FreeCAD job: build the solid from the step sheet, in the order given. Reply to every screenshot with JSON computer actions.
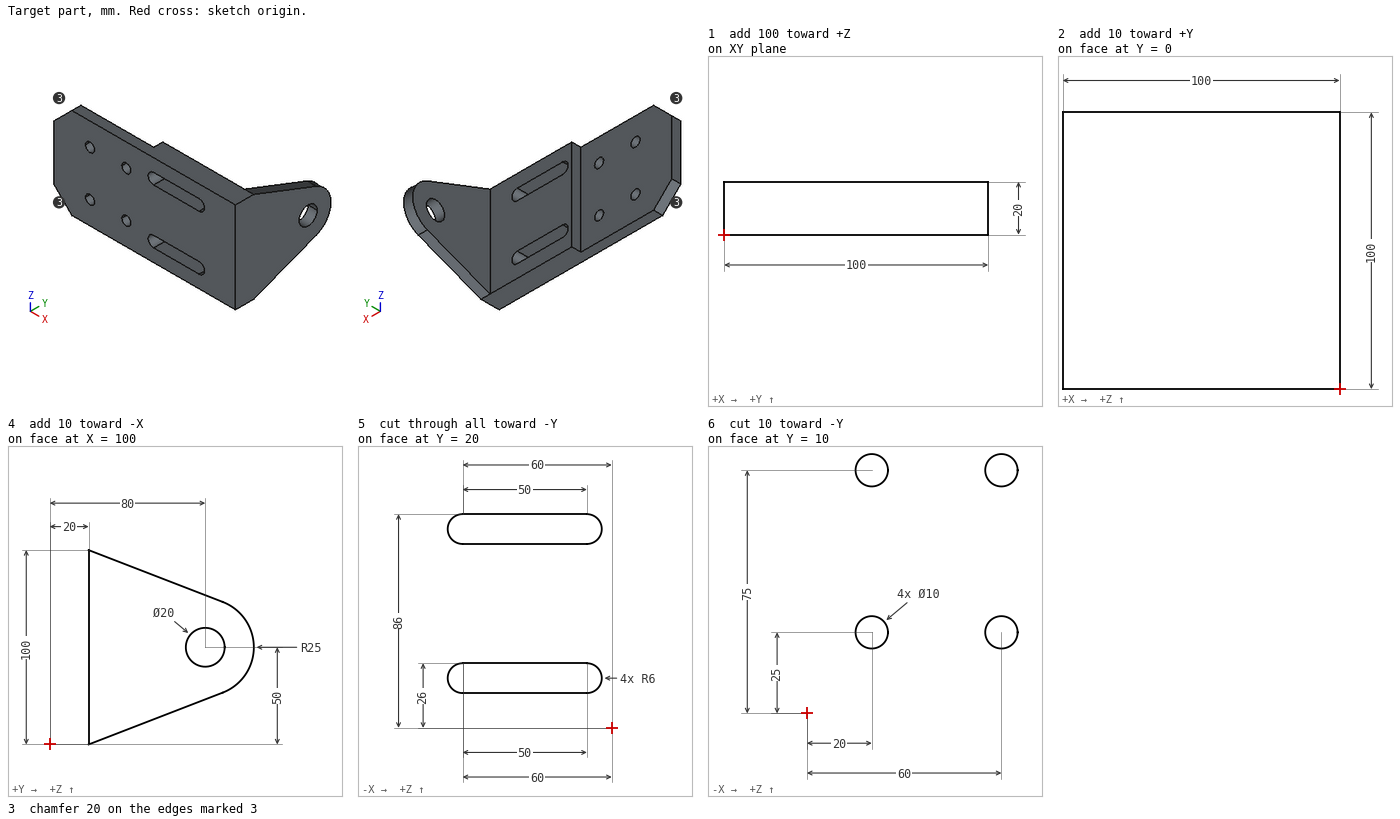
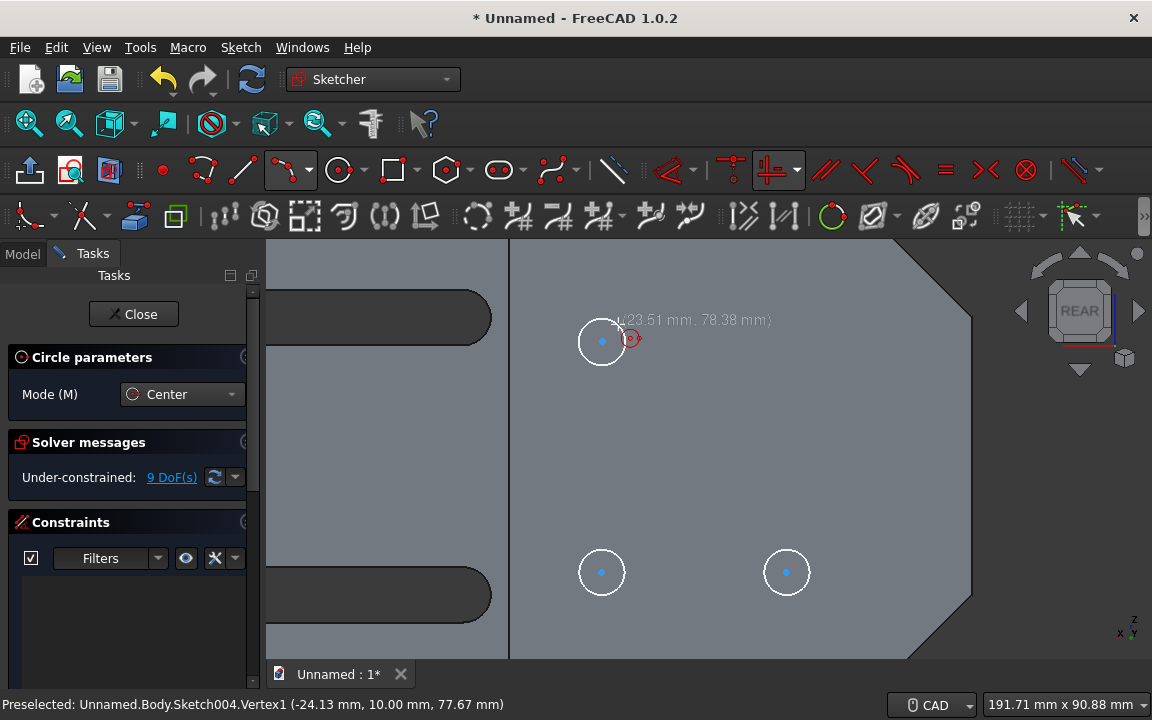
{"action": "left_click", "coordinate": [787, 341]}
{"action": "left_click", "coordinate": [803, 324]}
{"action": "key", "text": "Escape"}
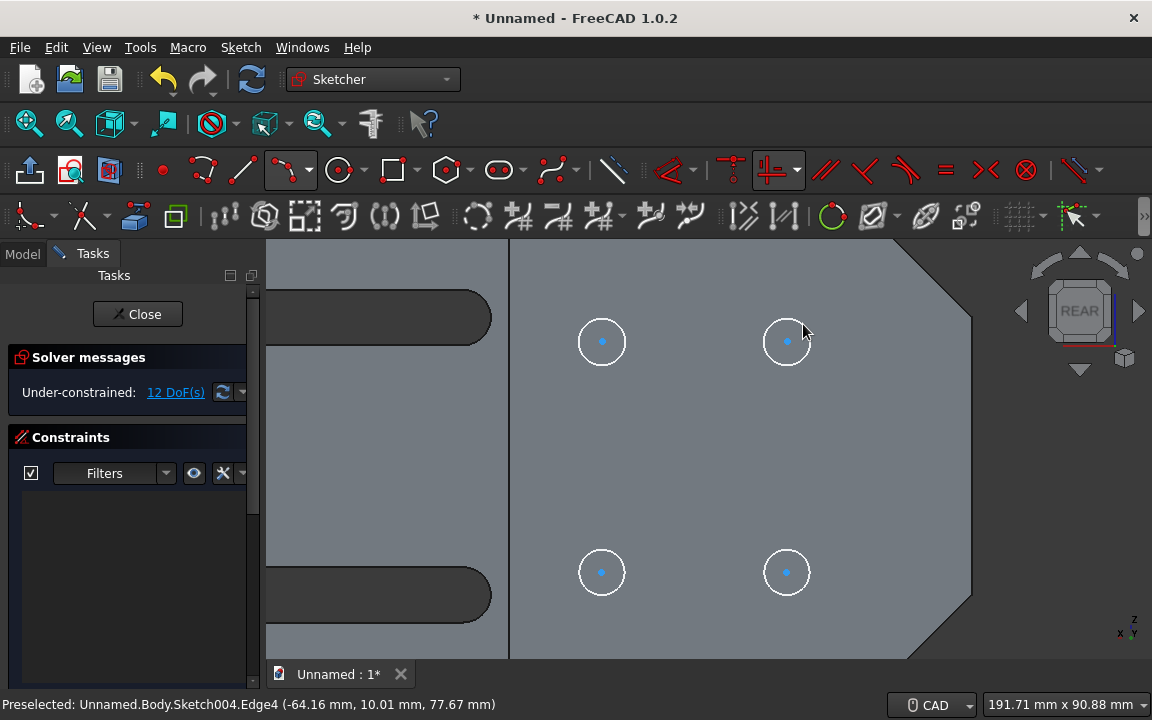
{"action": "left_click", "coordinate": [618, 556]}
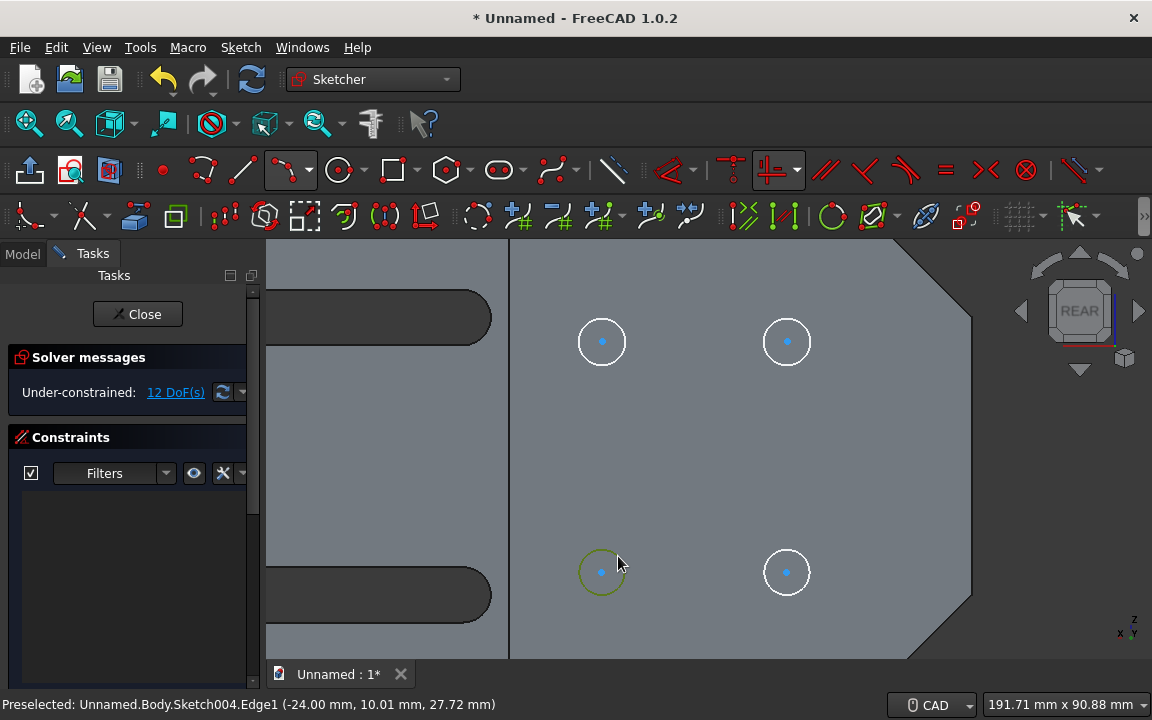
{"action": "left_click", "coordinate": [803, 556]}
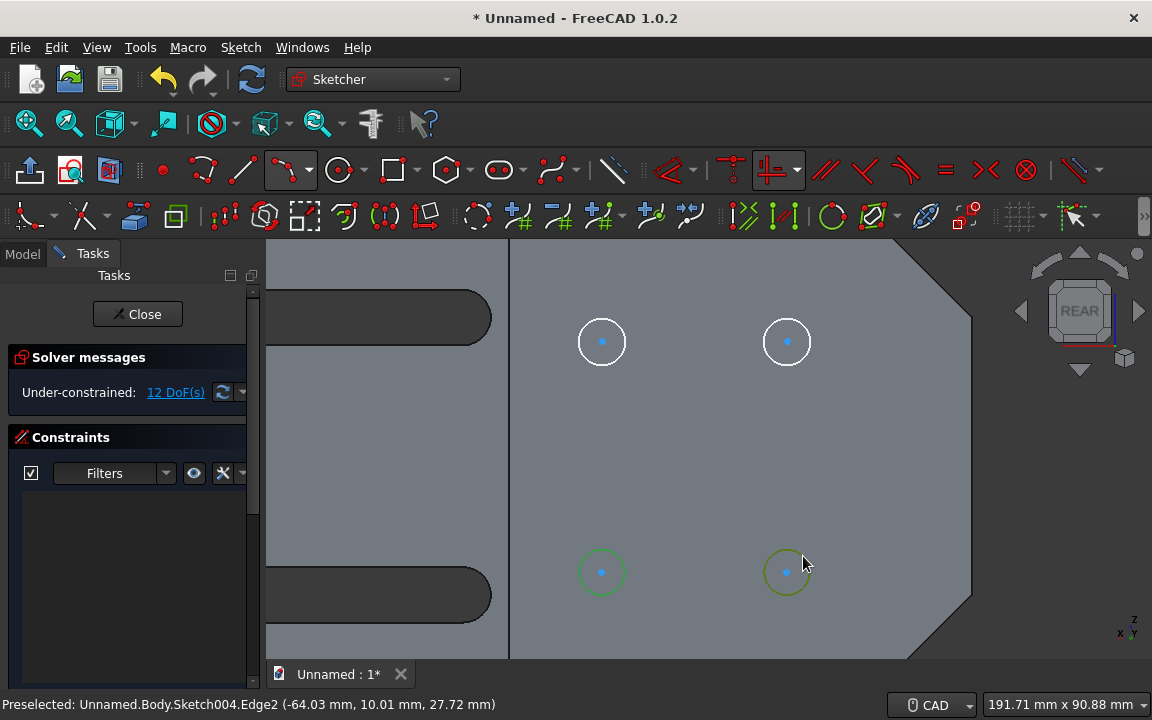
{"action": "left_click", "coordinate": [618, 325]}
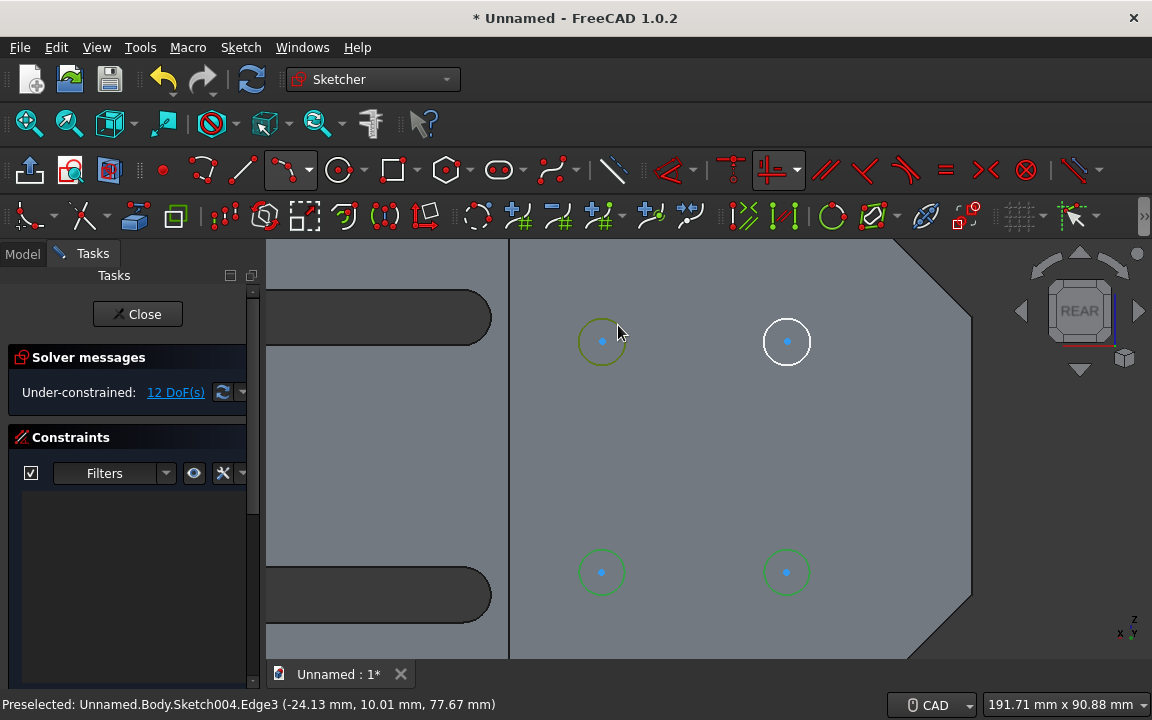
{"action": "left_click", "coordinate": [803, 325]}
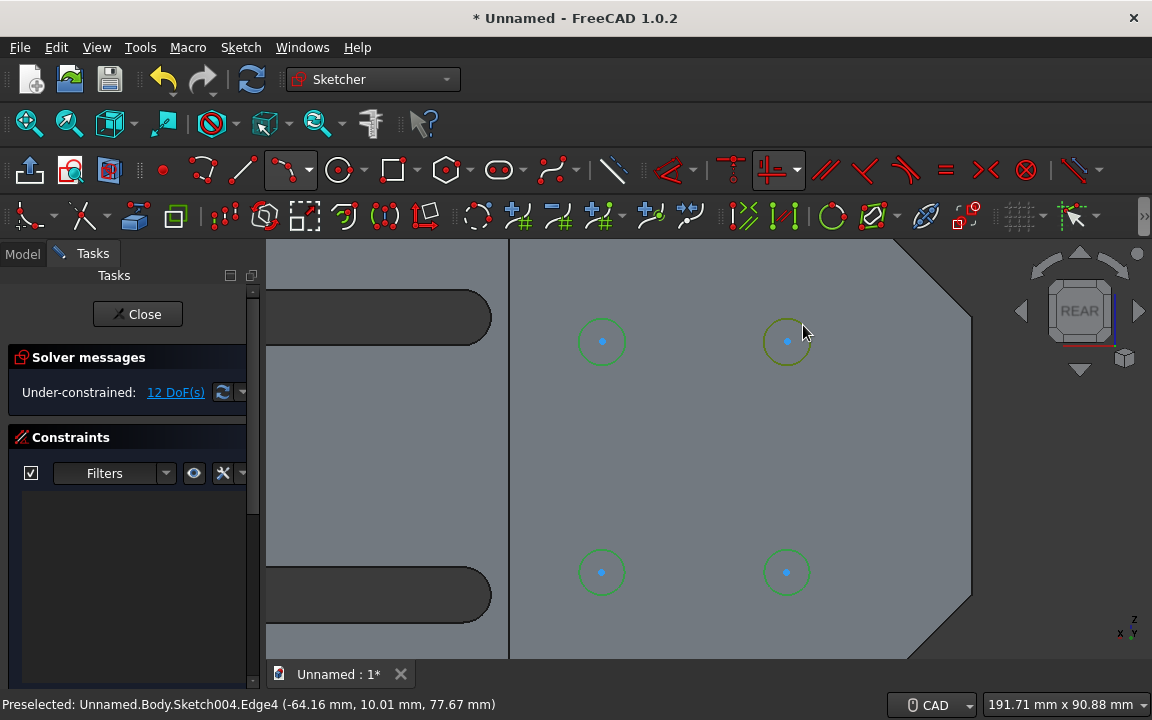
{"action": "left_click", "coordinate": [946, 170]}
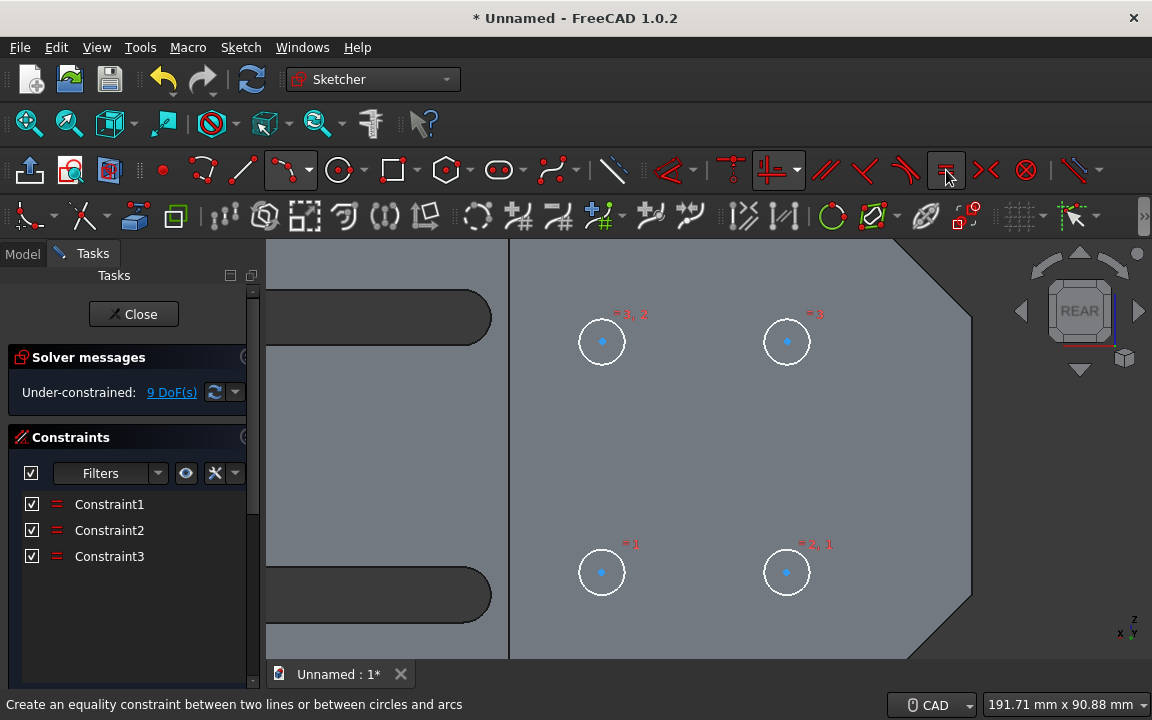
{"action": "left_click", "coordinate": [602, 572]}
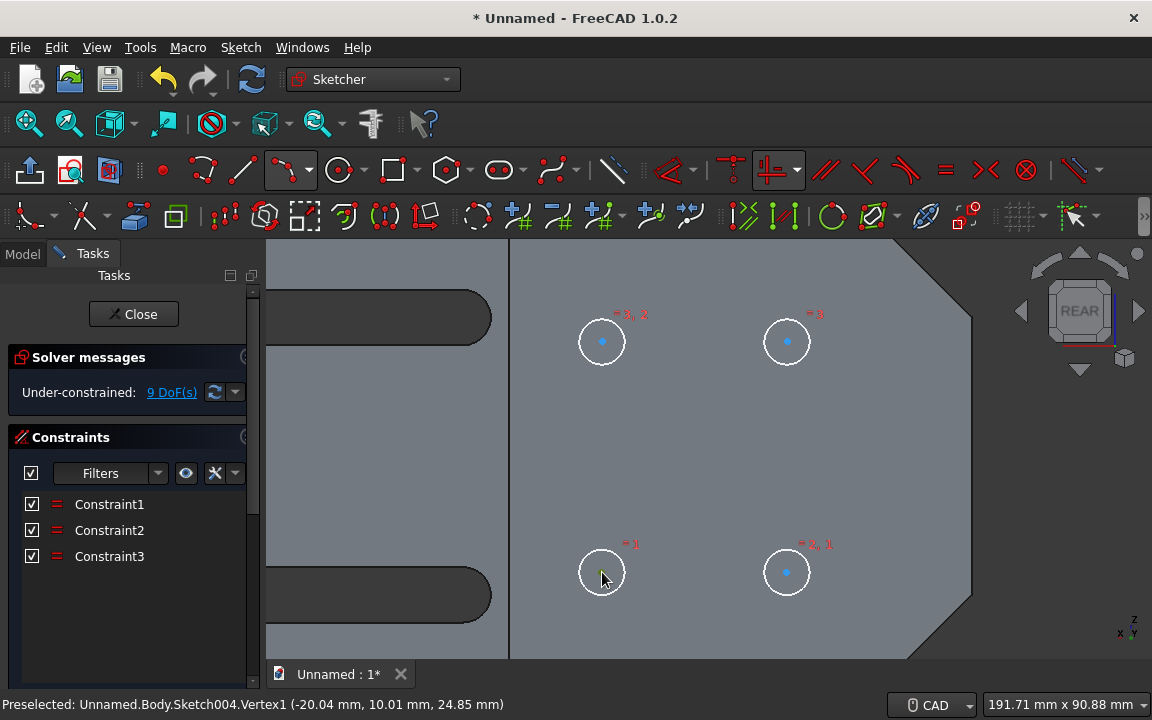
{"action": "left_click", "coordinate": [787, 572]}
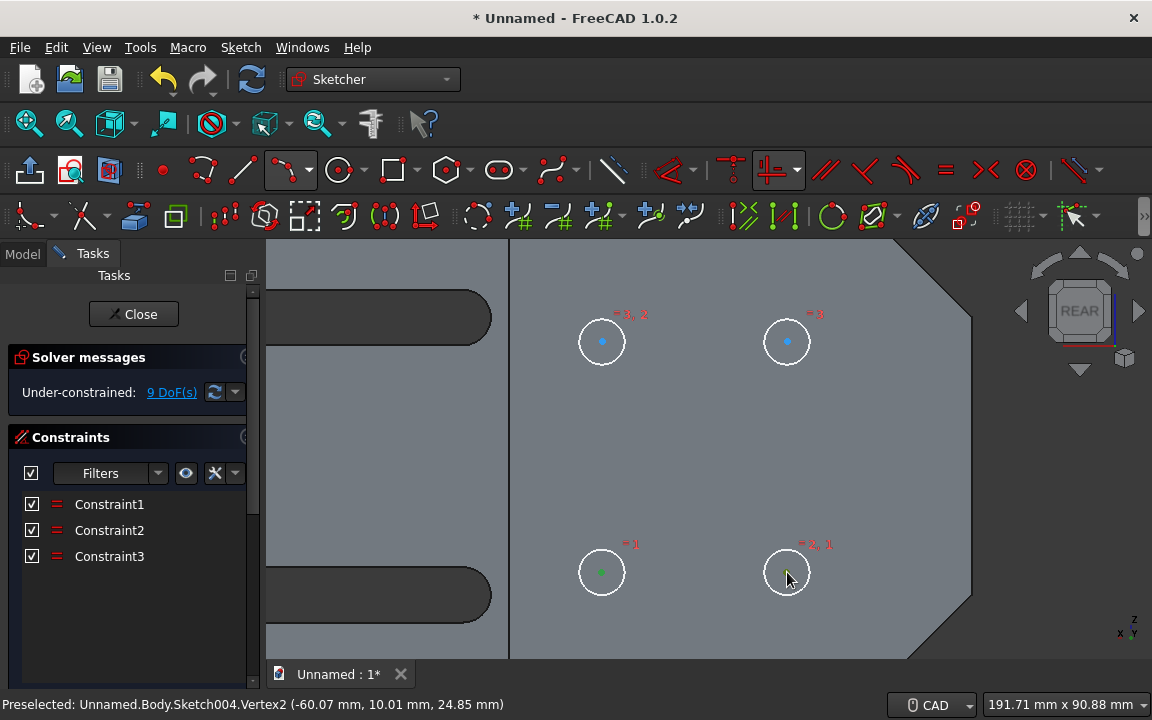
{"action": "key", "text": "h"}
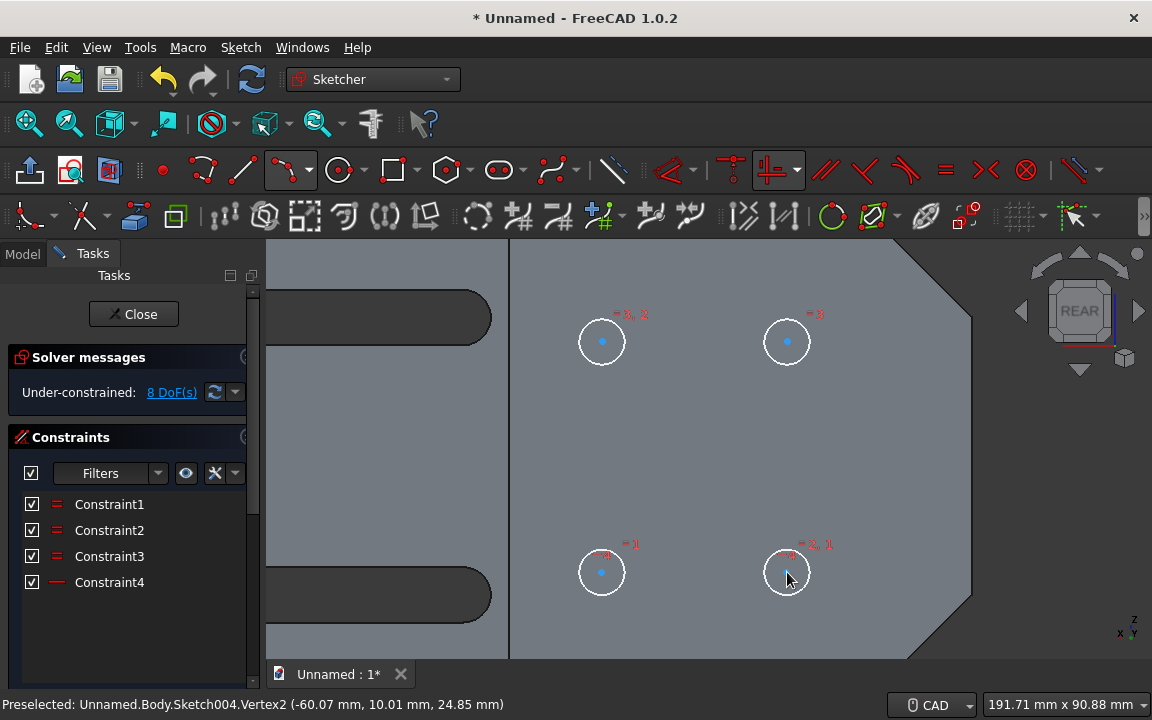
{"action": "left_click", "coordinate": [602, 572]}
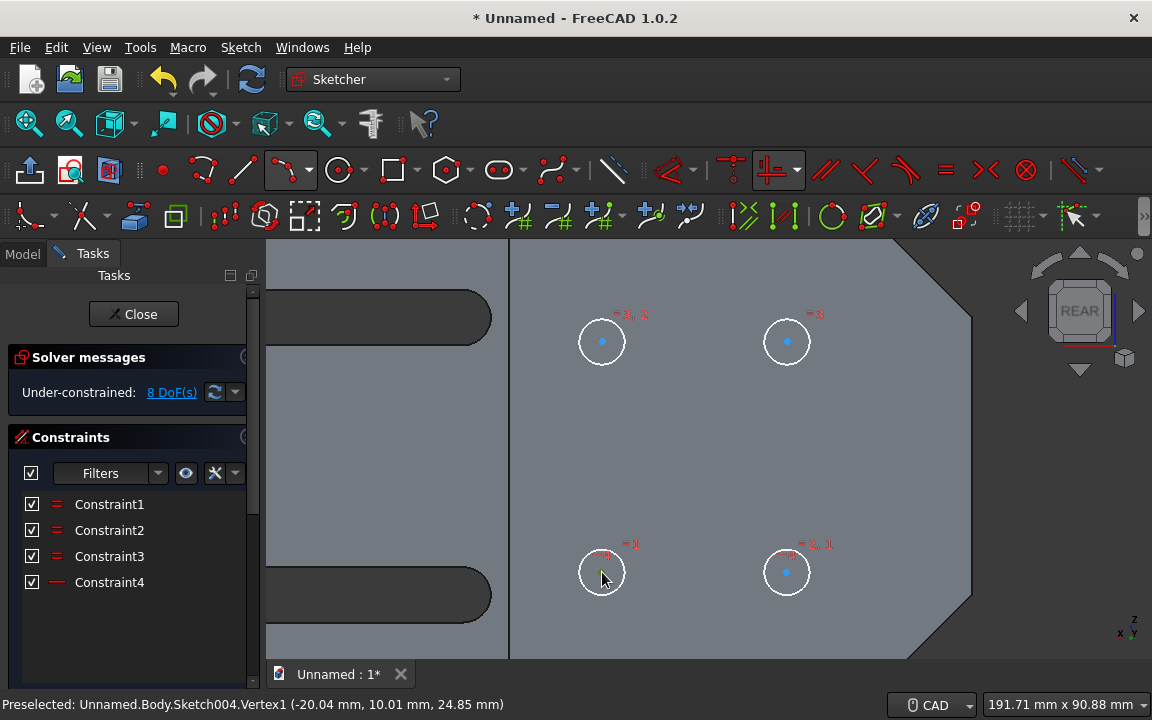
{"action": "left_click", "coordinate": [602, 342]}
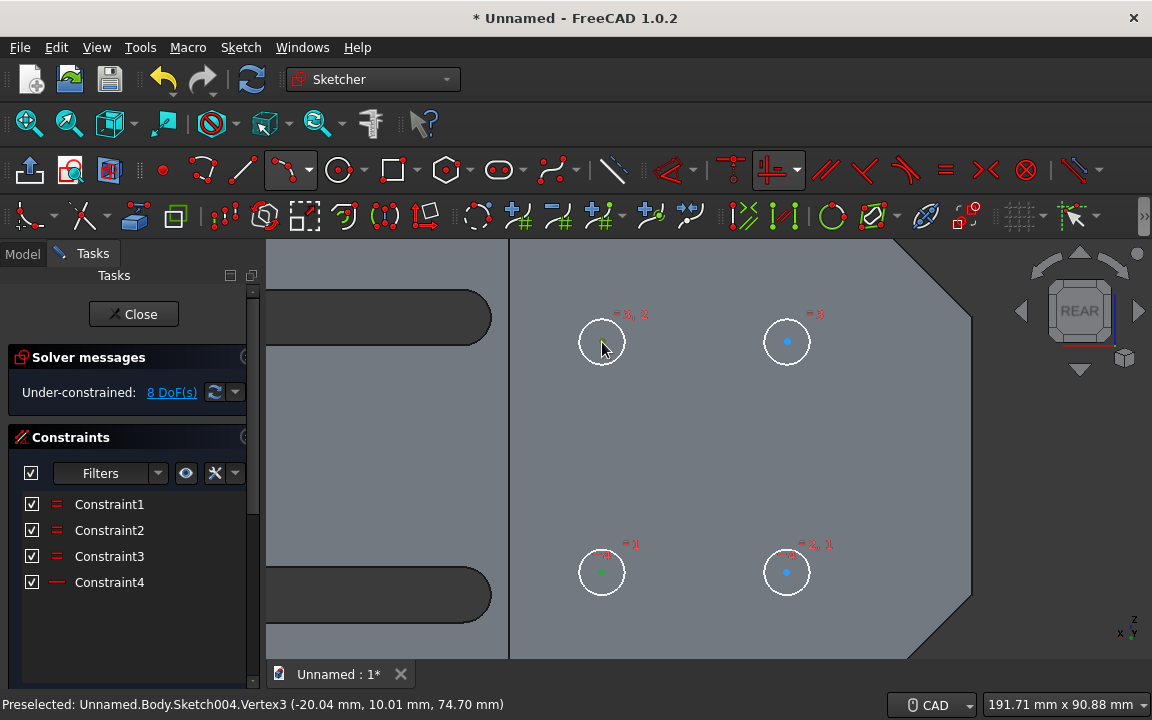
{"action": "left_click", "coordinate": [800, 170]}